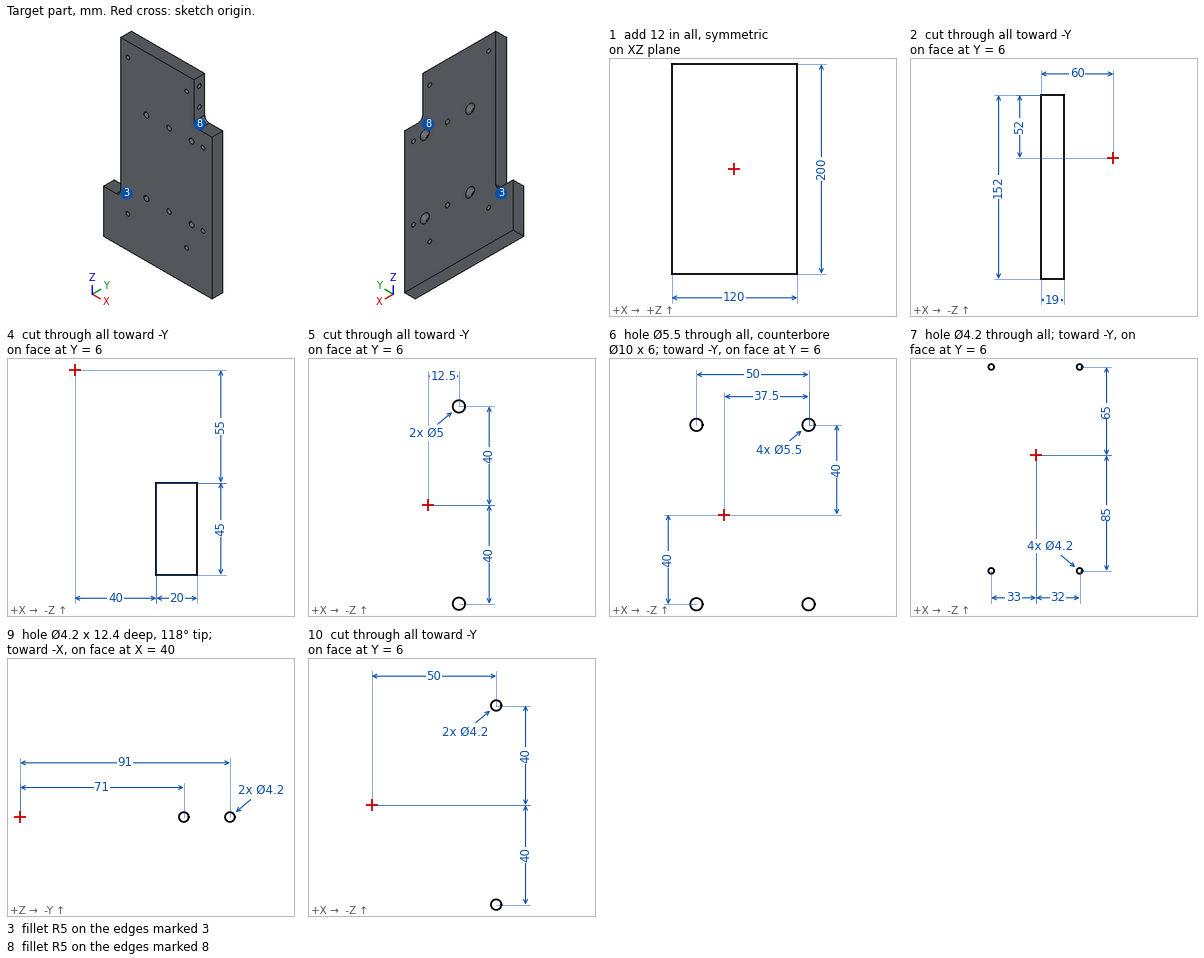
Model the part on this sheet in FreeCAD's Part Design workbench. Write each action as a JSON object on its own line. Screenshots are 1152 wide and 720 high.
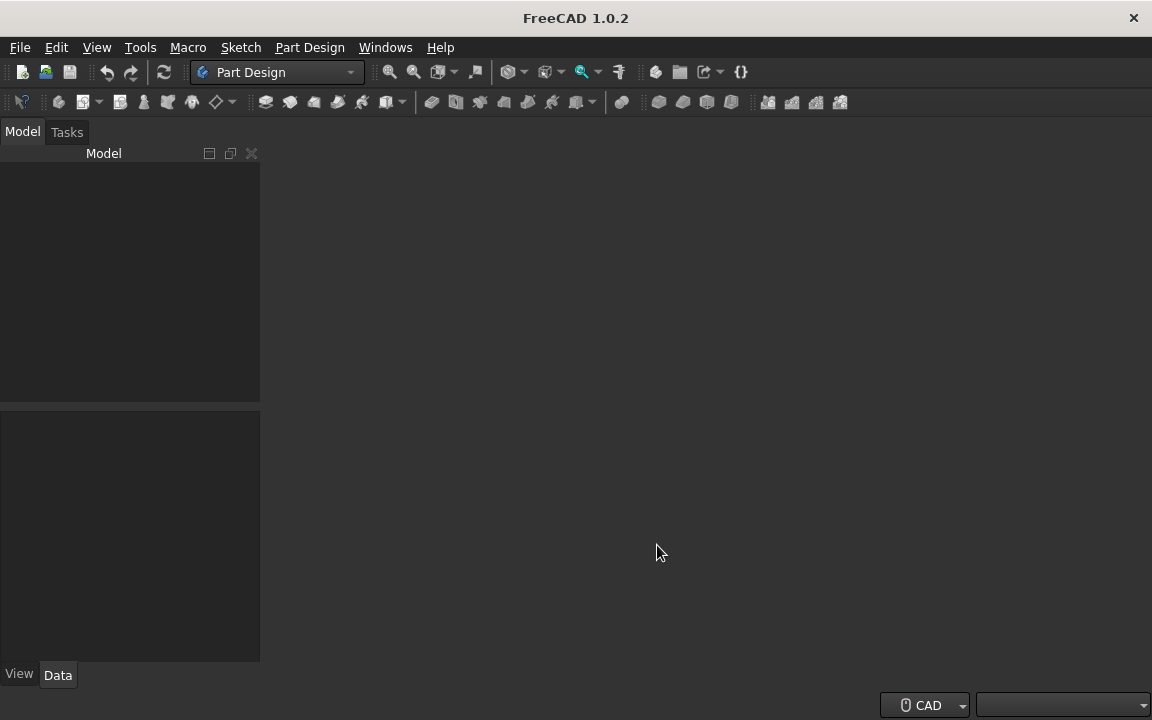
{"action": "left_click", "coordinate": [22, 72]}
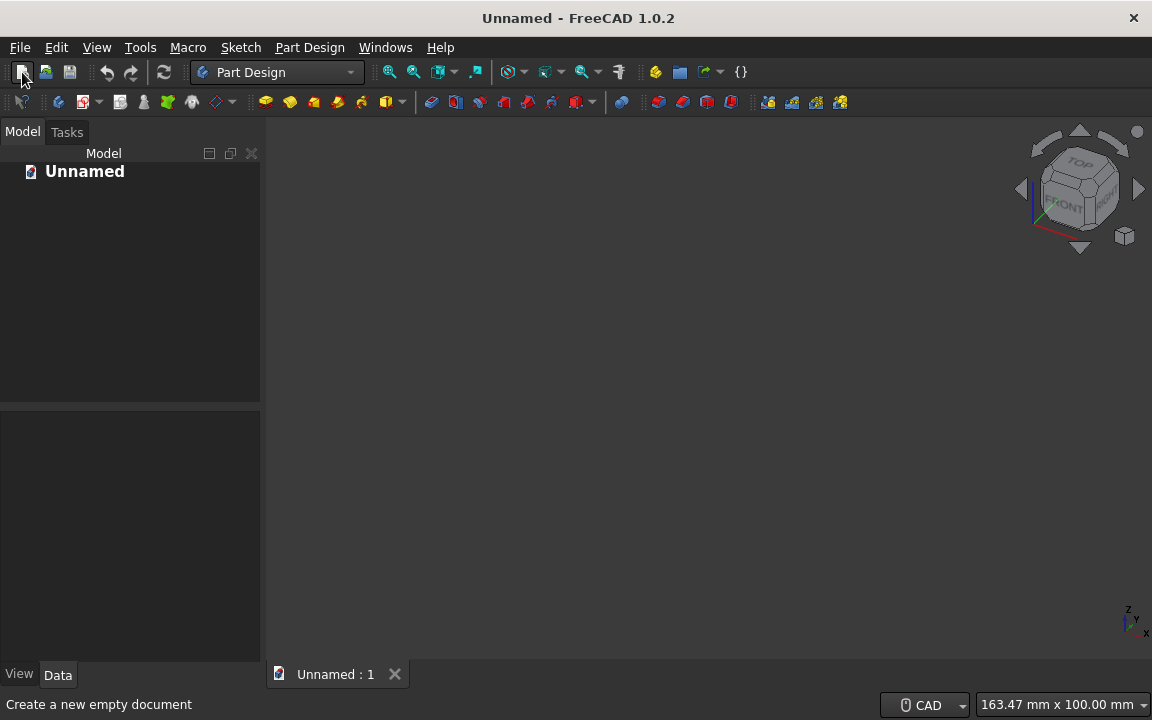
{"action": "left_click", "coordinate": [84, 102]}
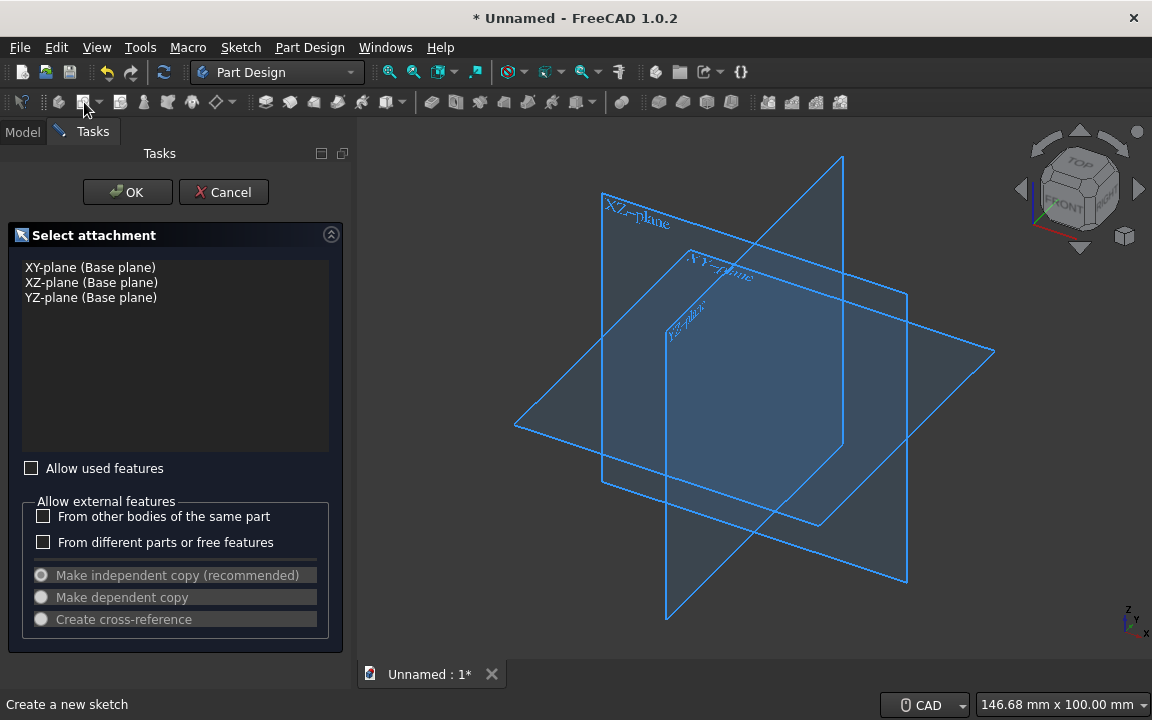
{"action": "left_click", "coordinate": [82, 282]}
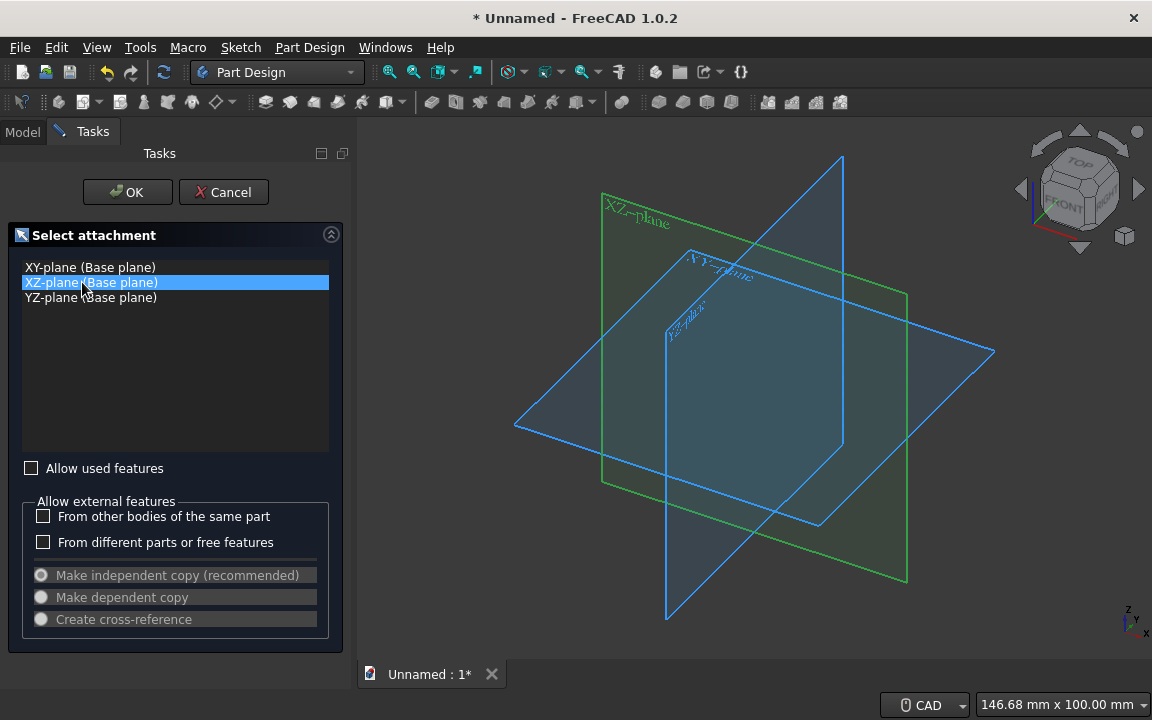
{"action": "left_click", "coordinate": [128, 192]}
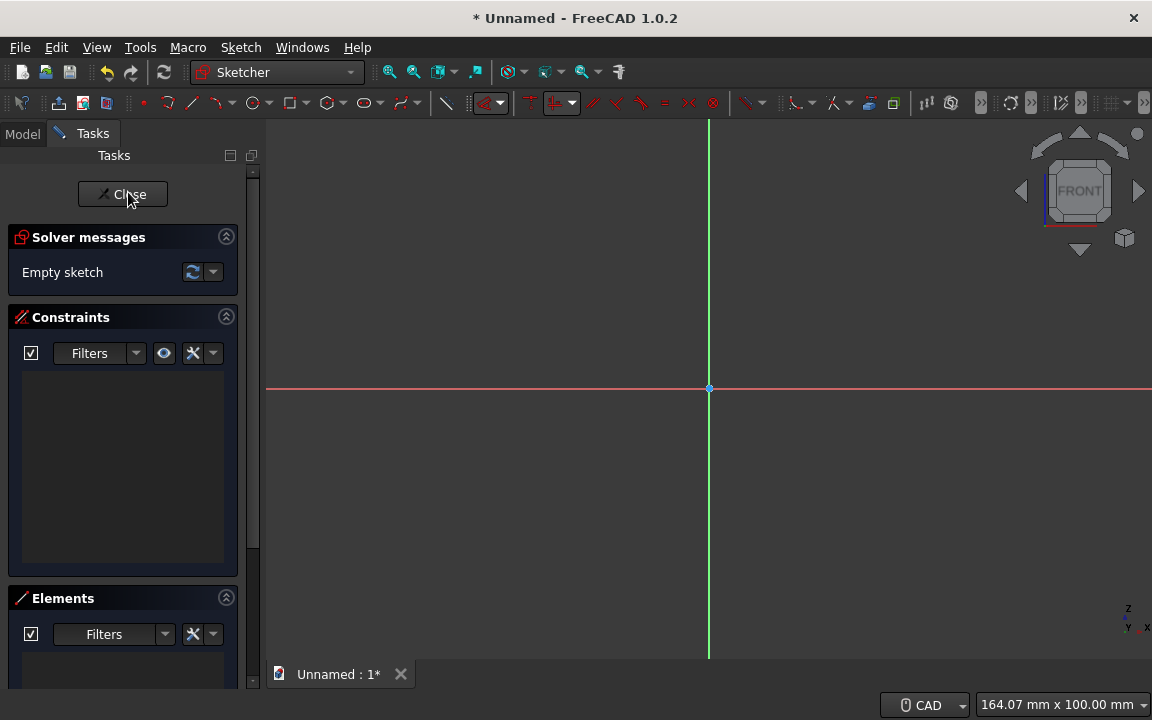
{"action": "scroll", "coordinate": [611, 389], "scroll_direction": "down", "scroll_amount": 6}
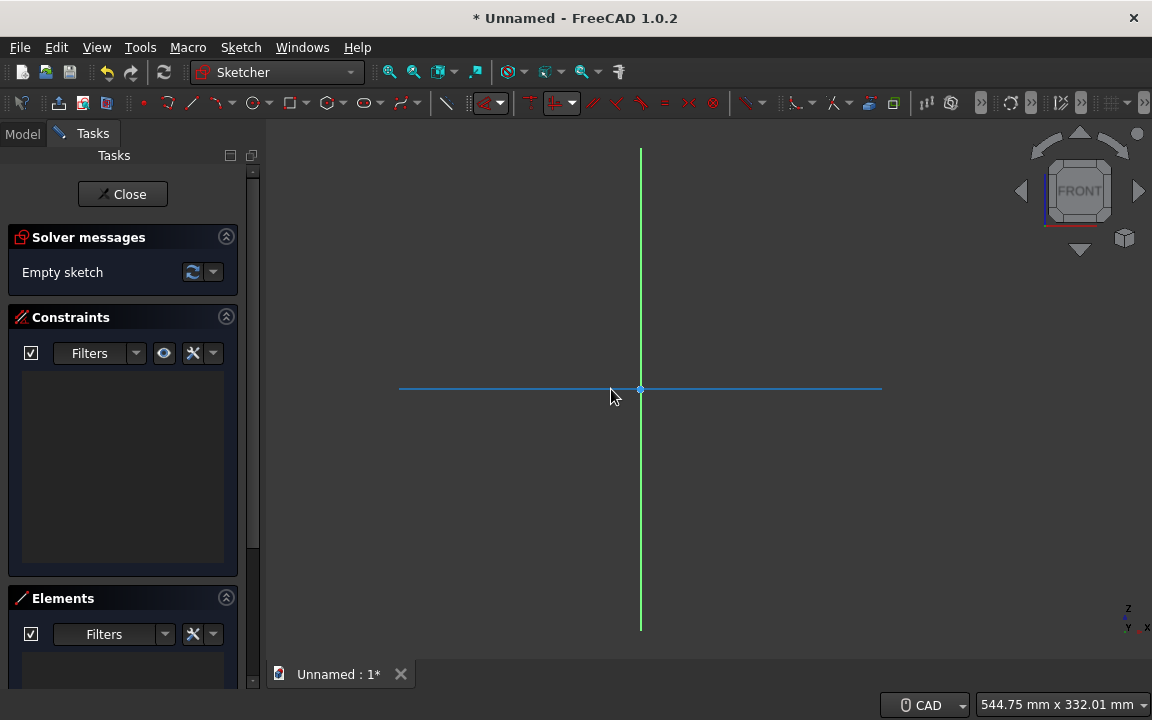
{"action": "left_click", "coordinate": [308, 104]}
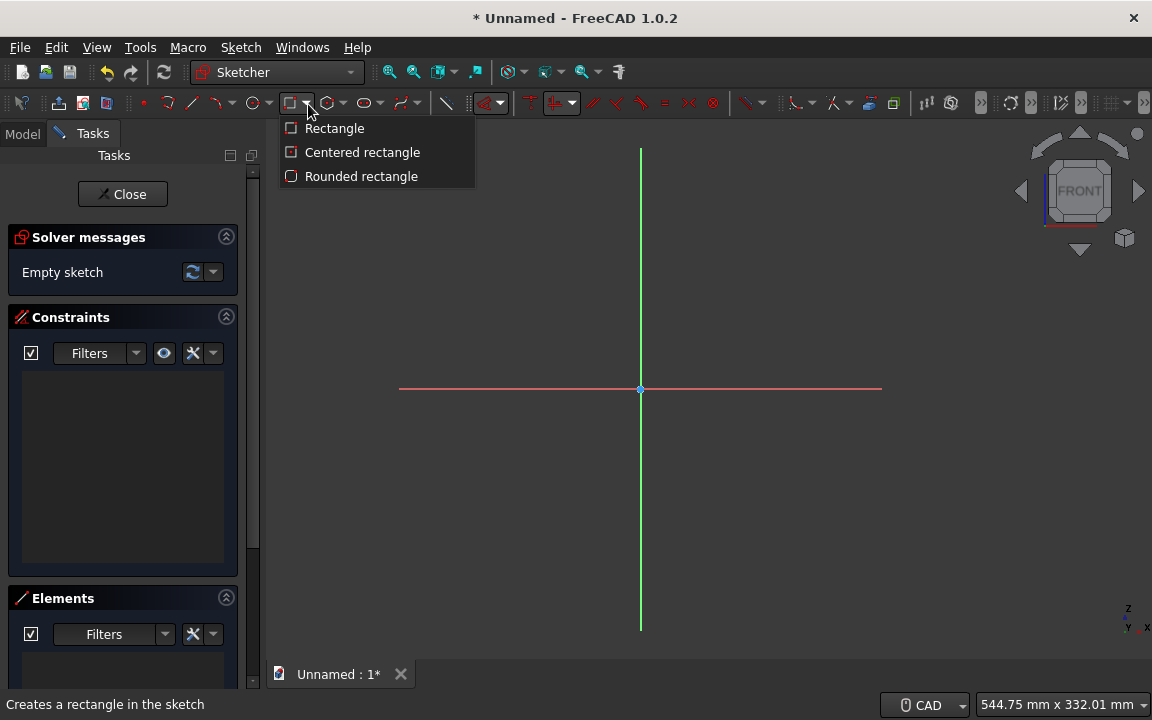
{"action": "left_click", "coordinate": [378, 152]}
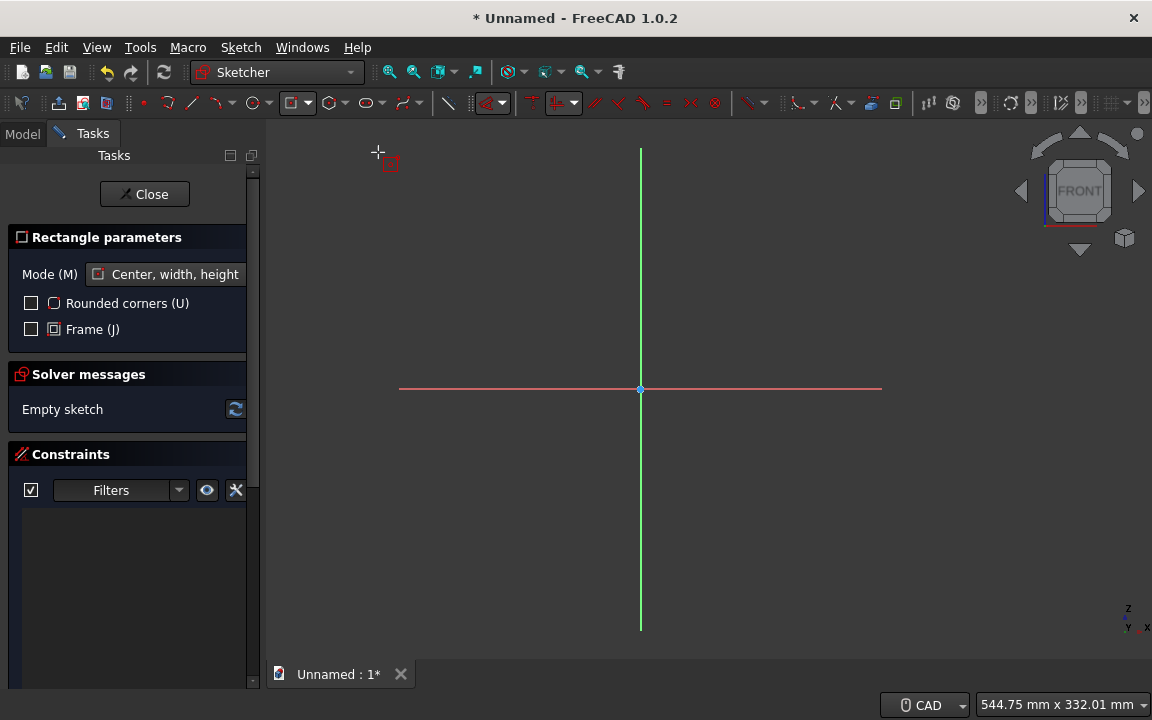
{"action": "left_click", "coordinate": [641, 389]}
{"action": "left_click", "coordinate": [738, 227]}
{"action": "key", "text": "Escape"}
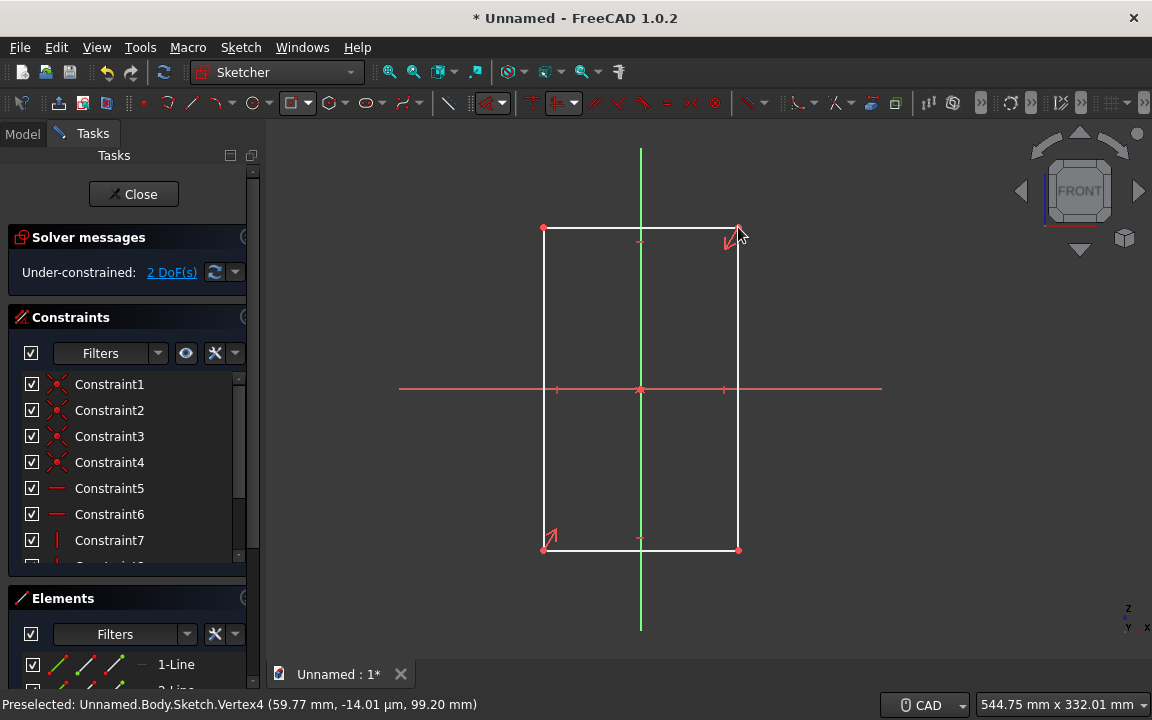
{"action": "left_click", "coordinate": [602, 551]}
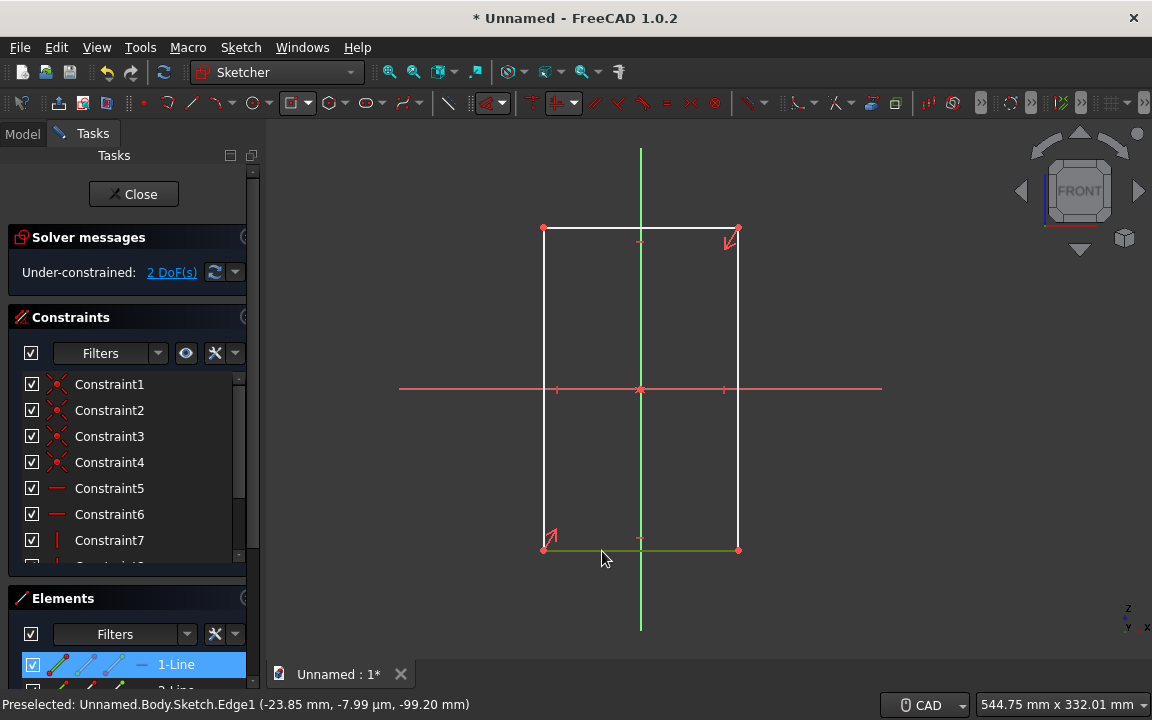
{"action": "key", "text": "l"}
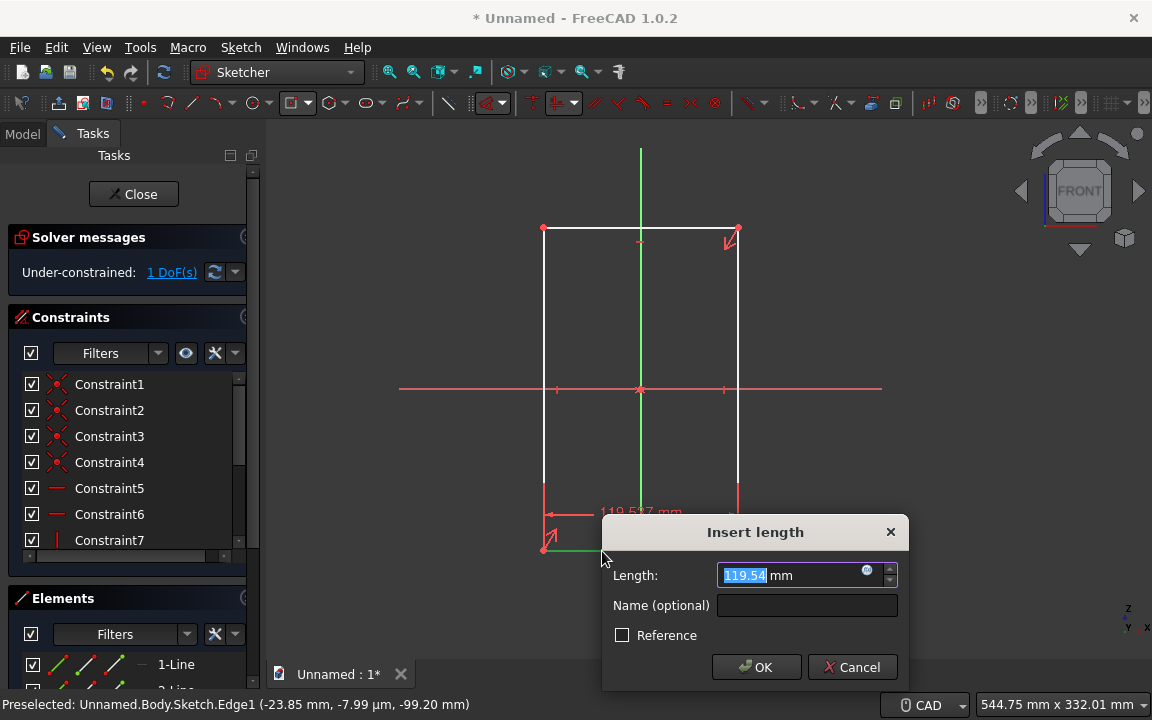
{"action": "type", "text": "120"}
{"action": "key", "text": "Return"}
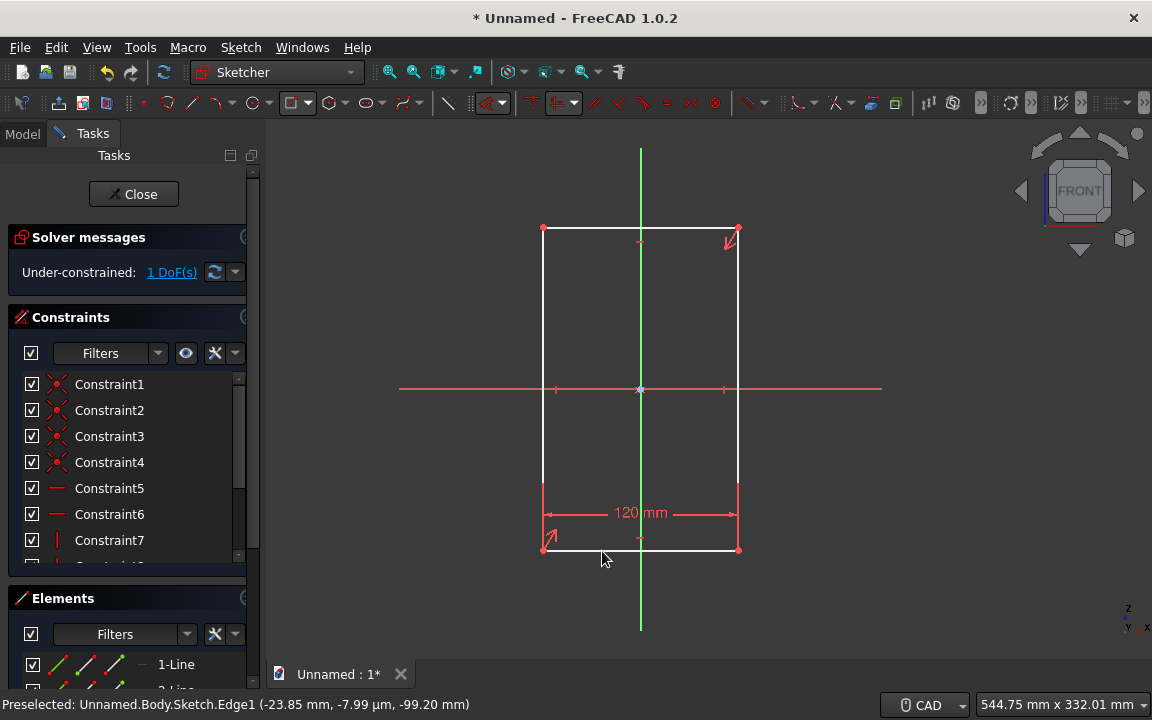
{"action": "left_click", "coordinate": [738, 454]}